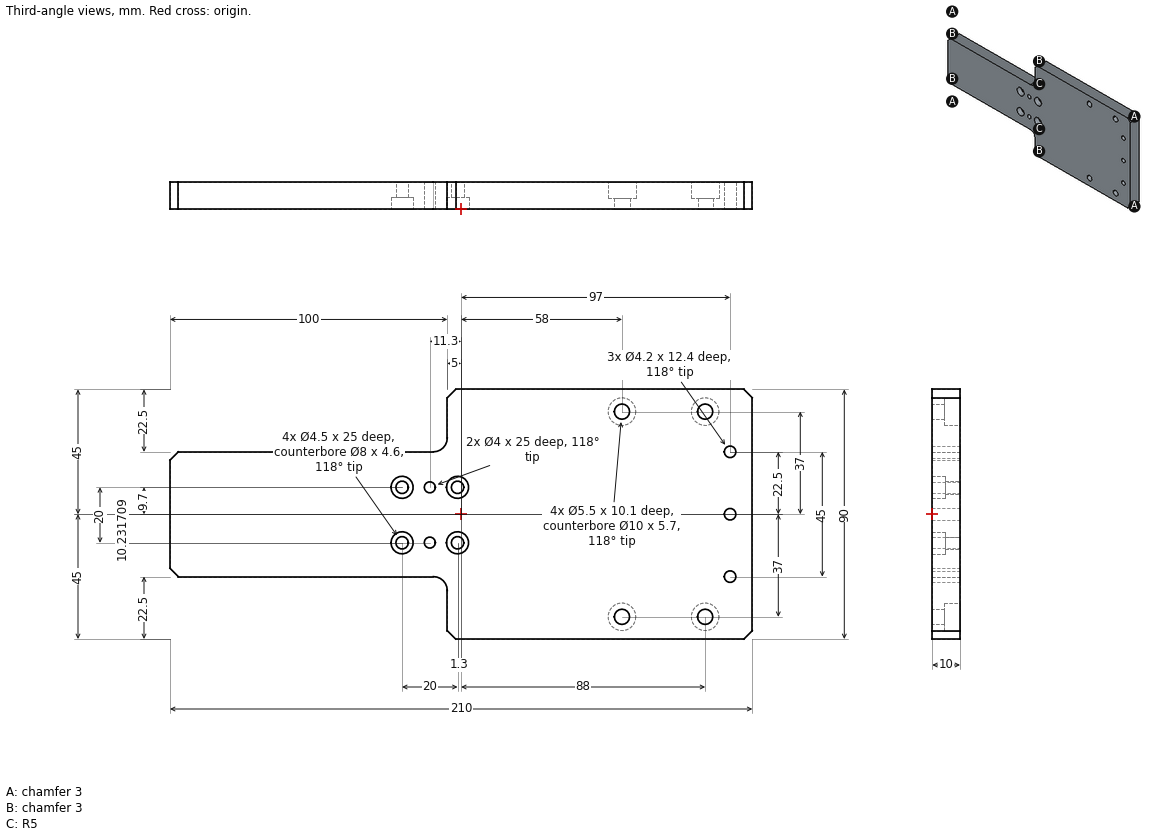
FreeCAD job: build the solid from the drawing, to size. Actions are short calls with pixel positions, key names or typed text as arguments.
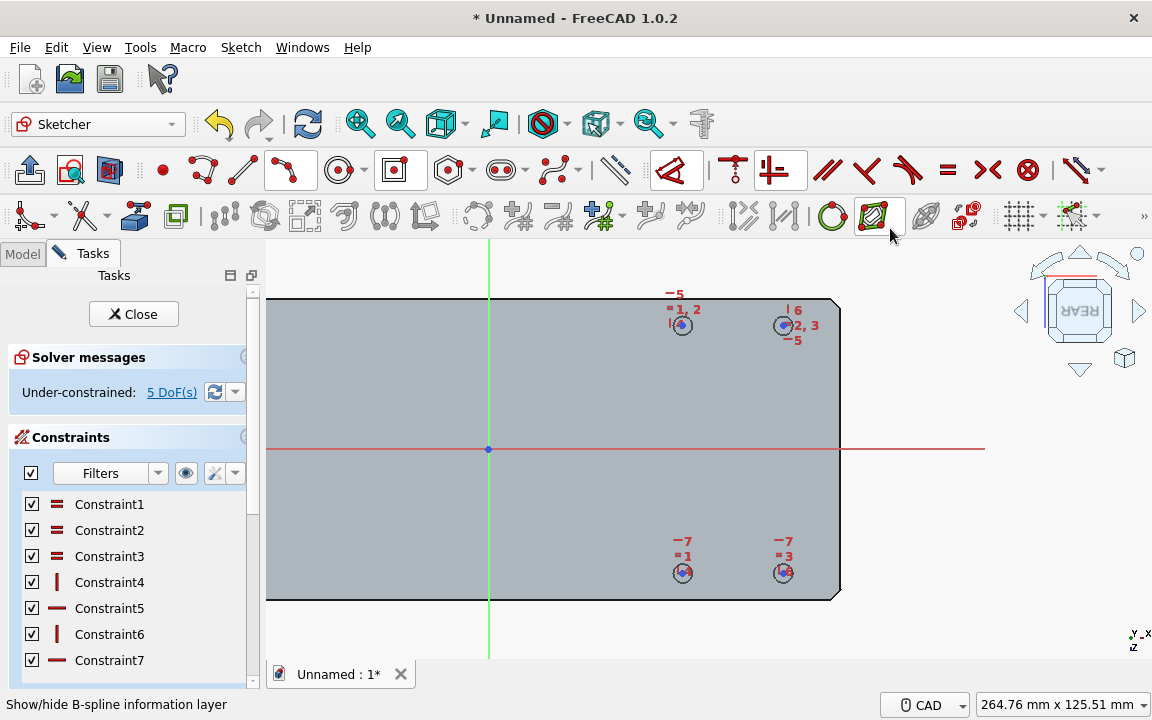
scroll(689, 567, up, 4)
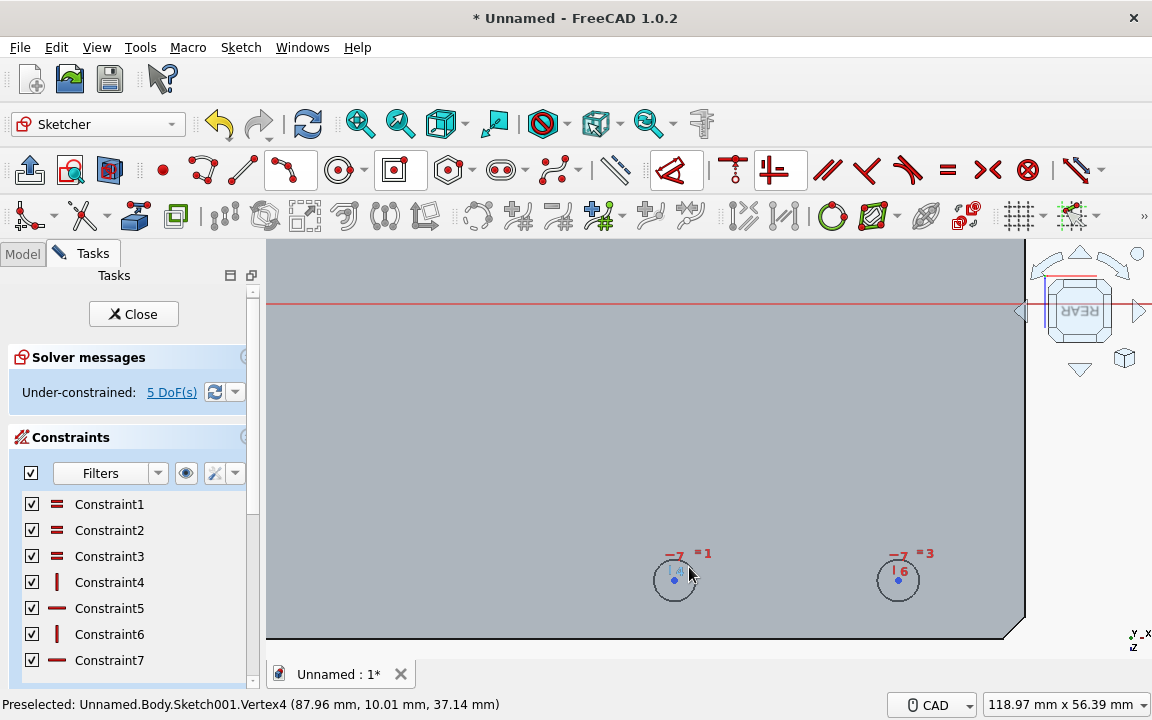
click(689, 566)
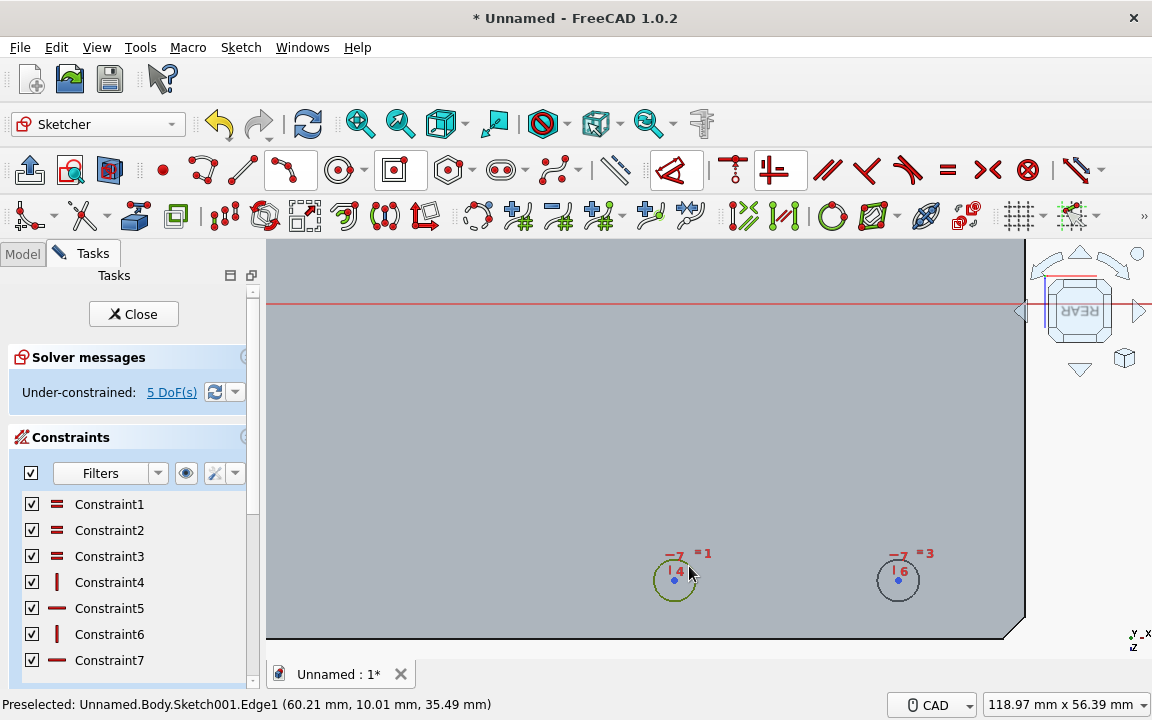
click(698, 170)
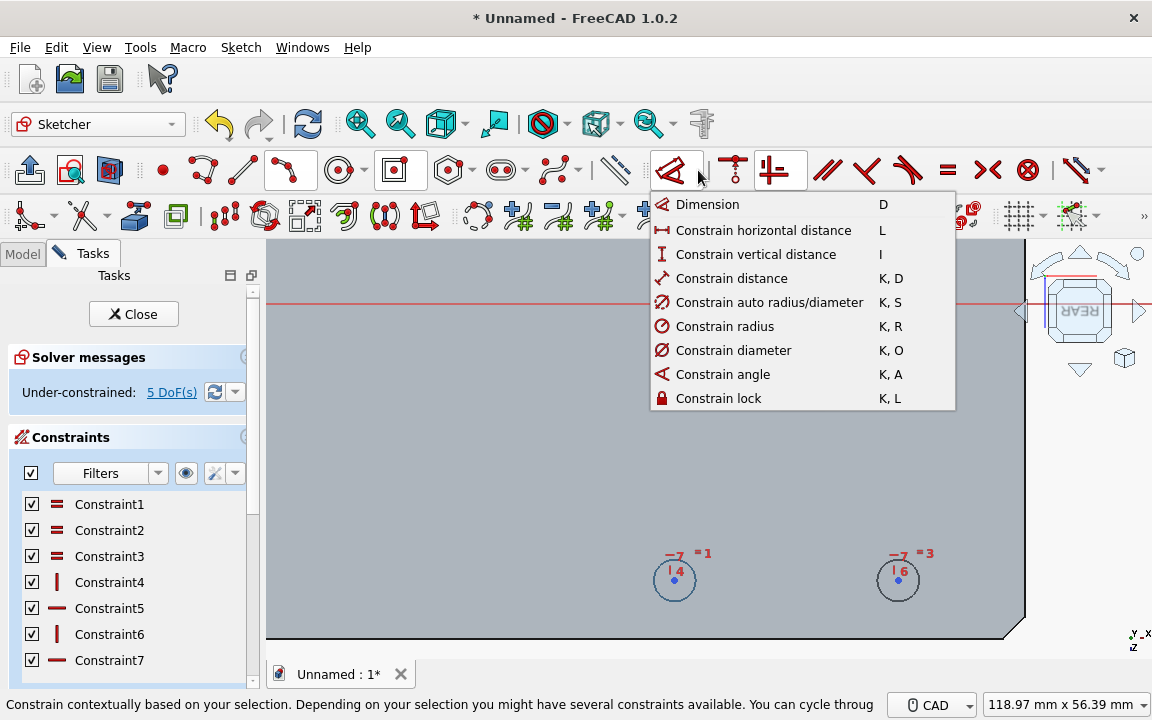
click(803, 350)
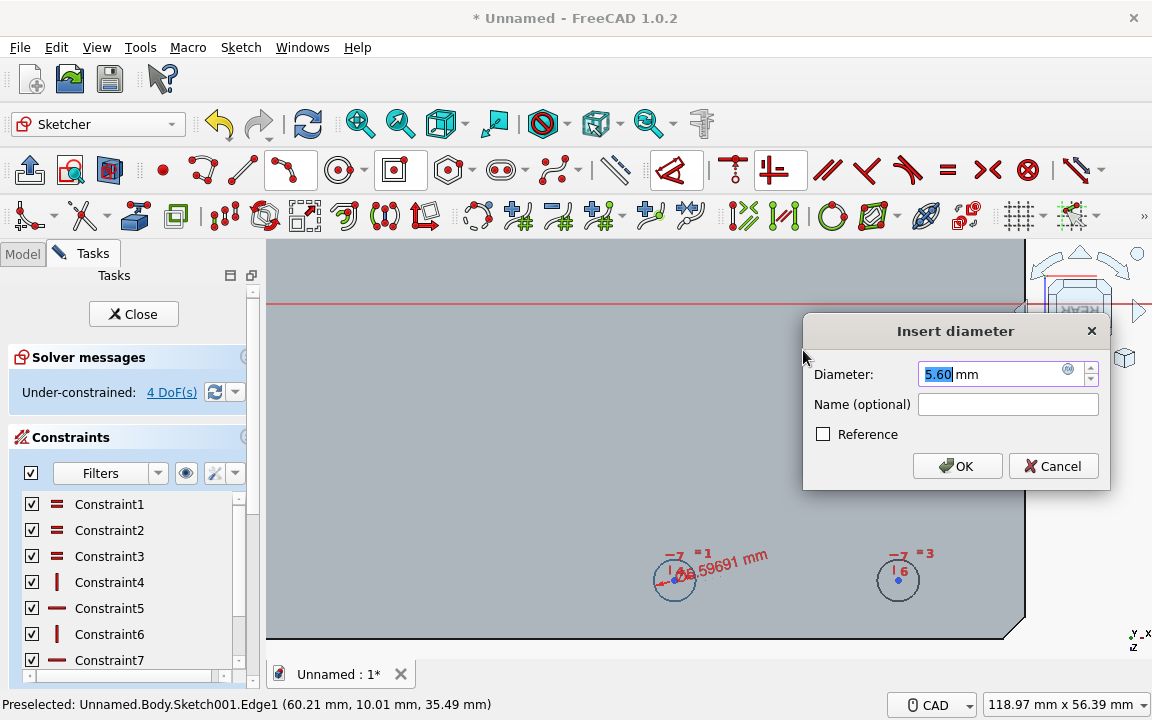
text(5.5)
key(Return)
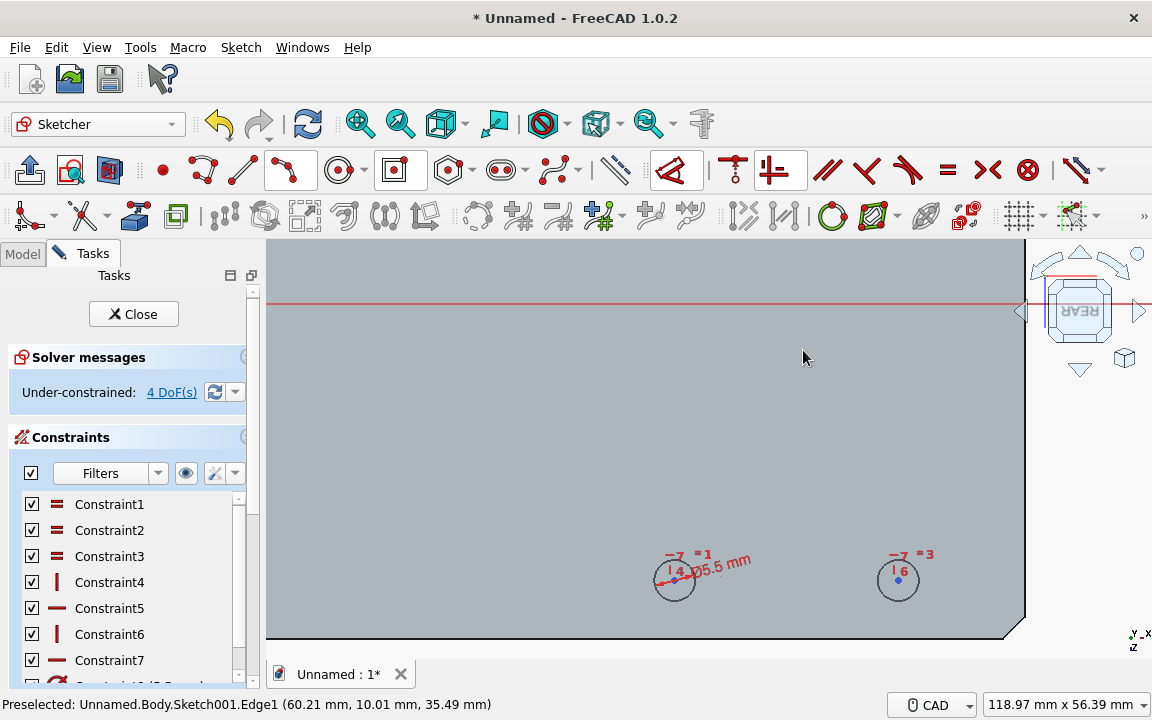
click(675, 581)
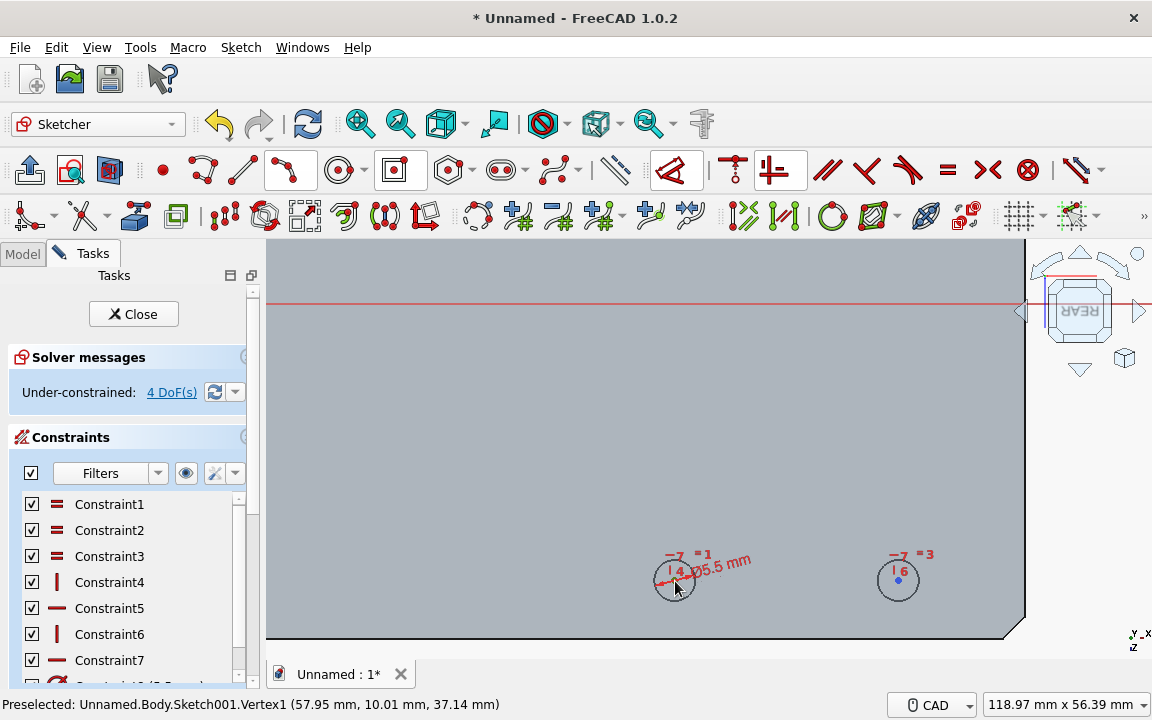
click(698, 170)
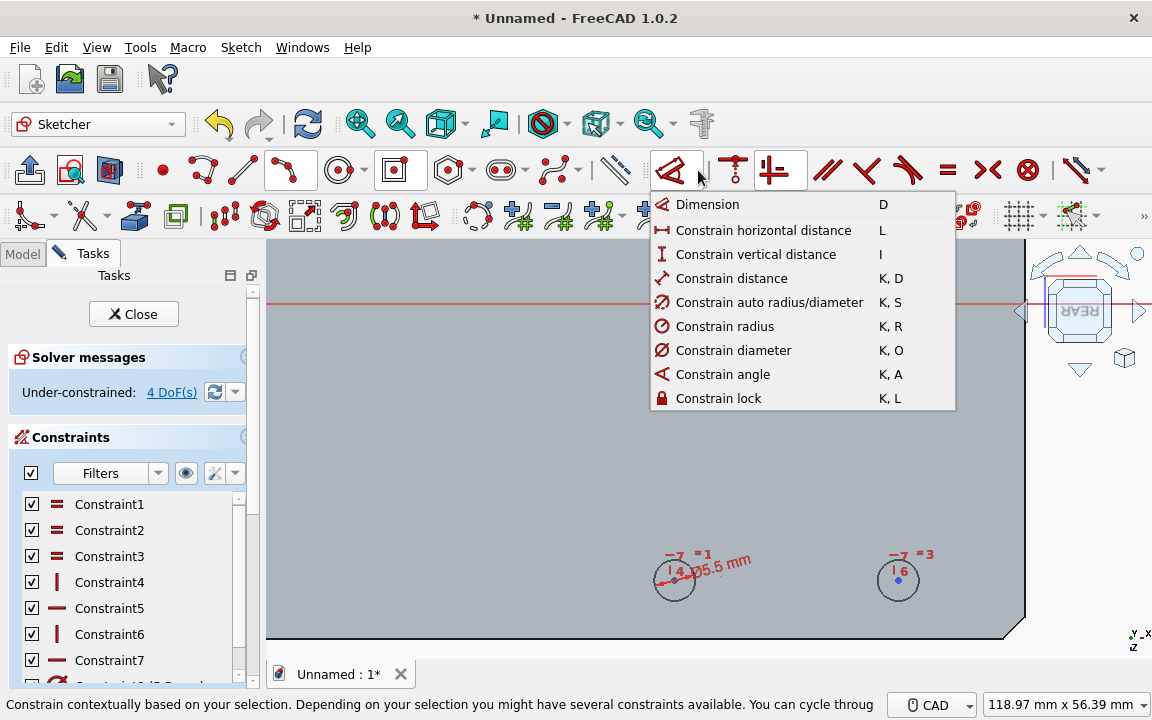
click(803, 230)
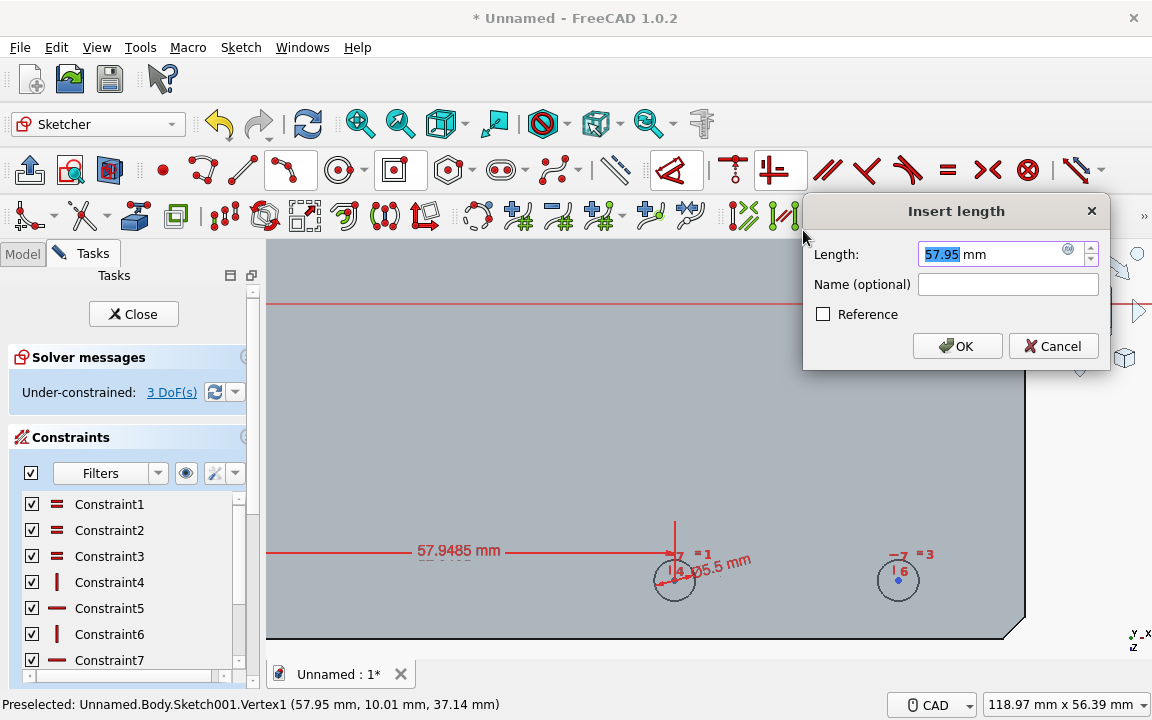
text(58)
key(Return)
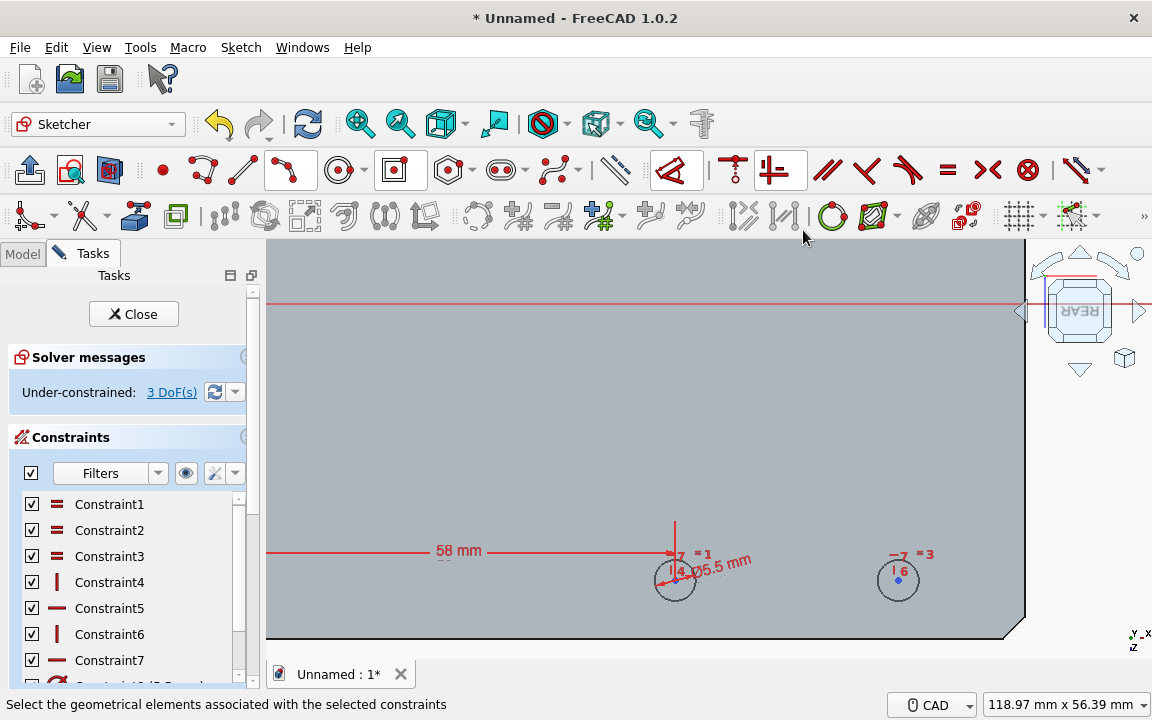
click(675, 581)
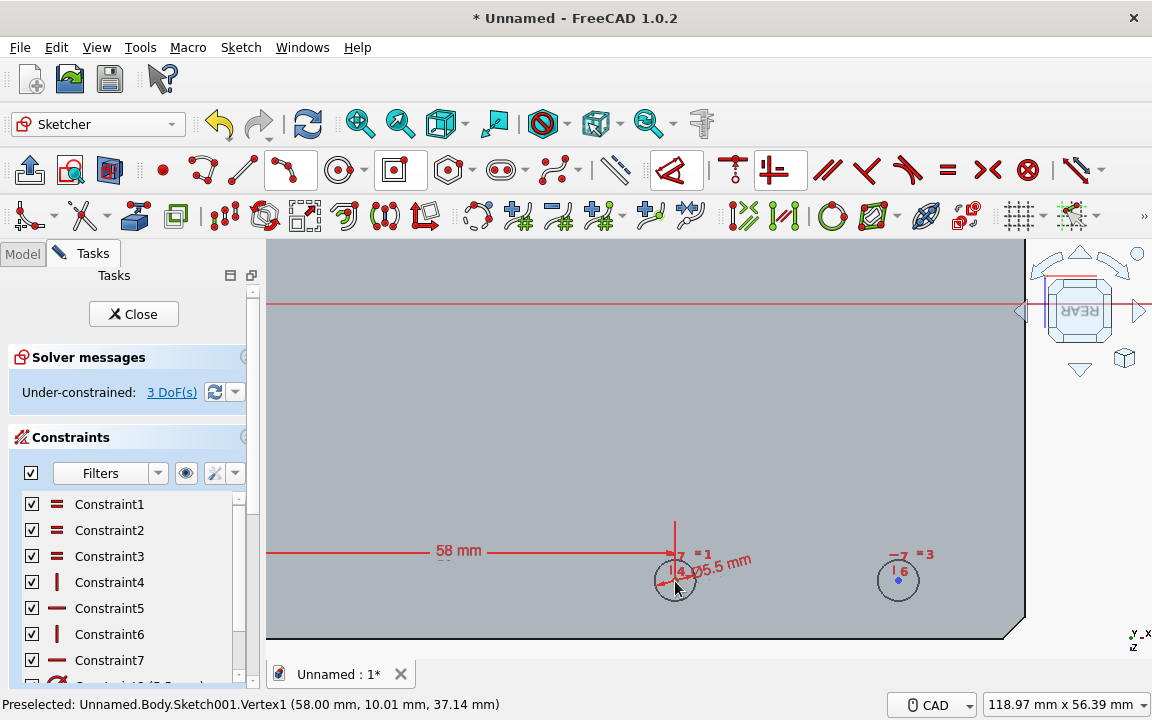
click(698, 170)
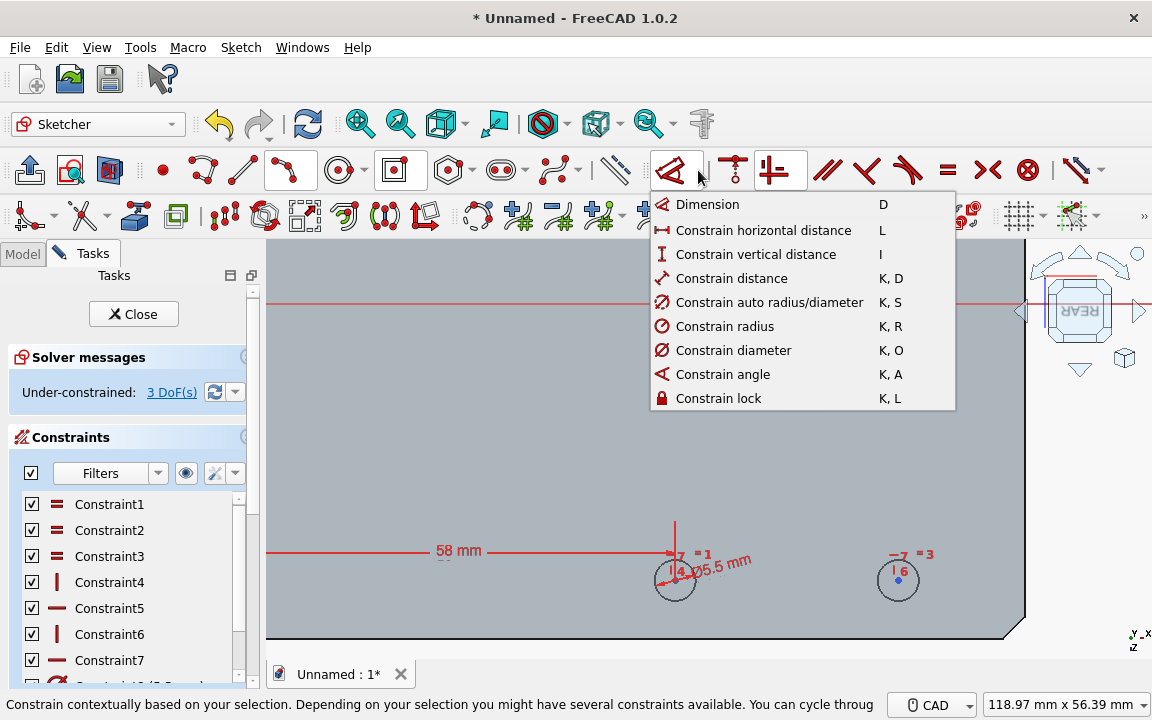
click(803, 254)